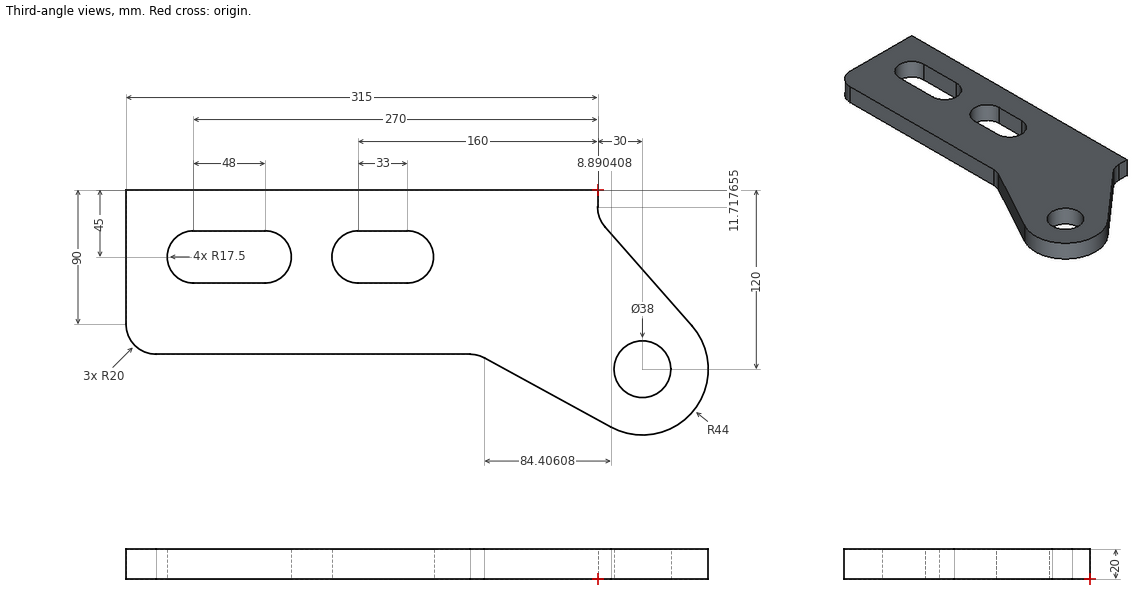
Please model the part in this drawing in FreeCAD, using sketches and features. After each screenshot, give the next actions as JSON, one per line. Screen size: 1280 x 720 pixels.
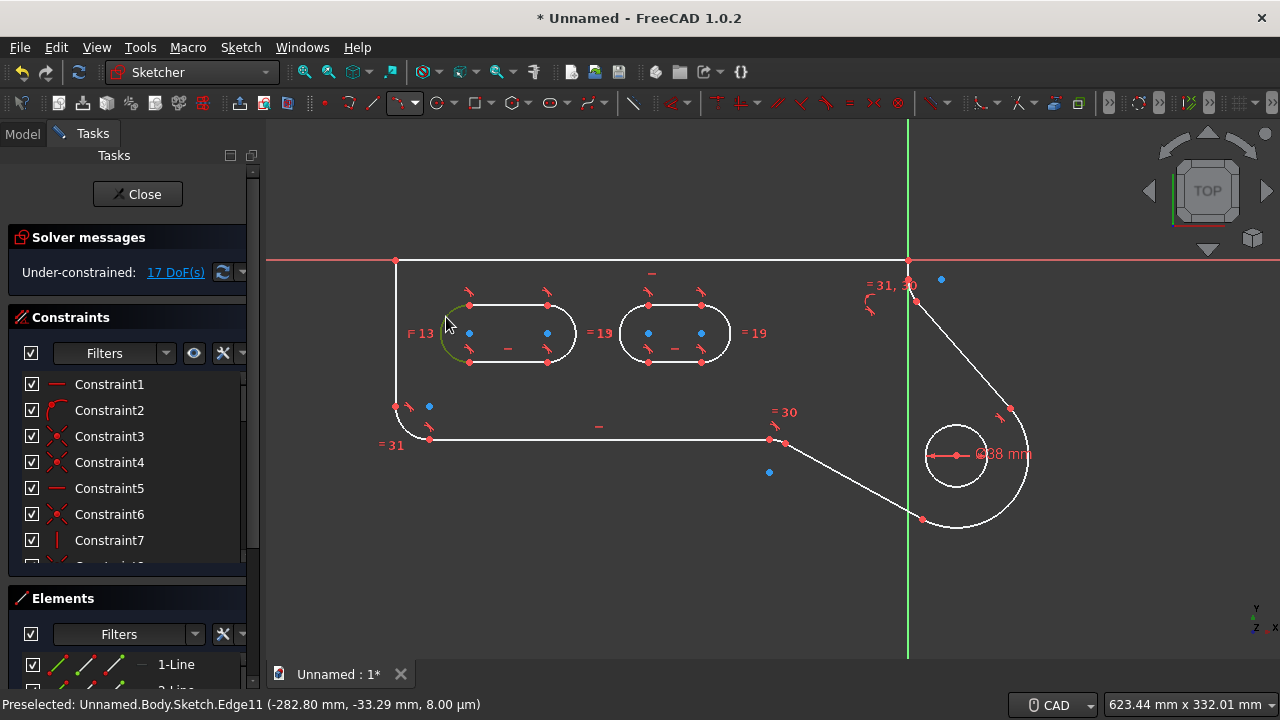
{"action": "left_click", "coordinate": [625, 317]}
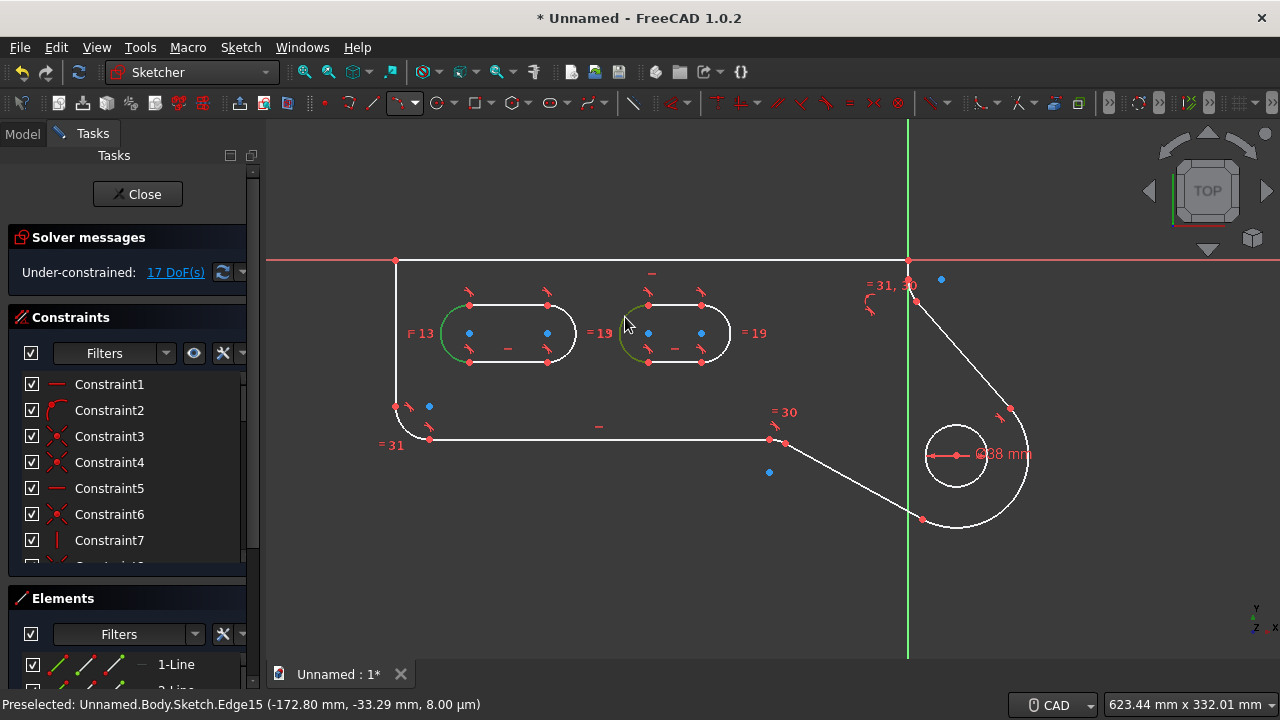
{"action": "left_click", "coordinate": [850, 104]}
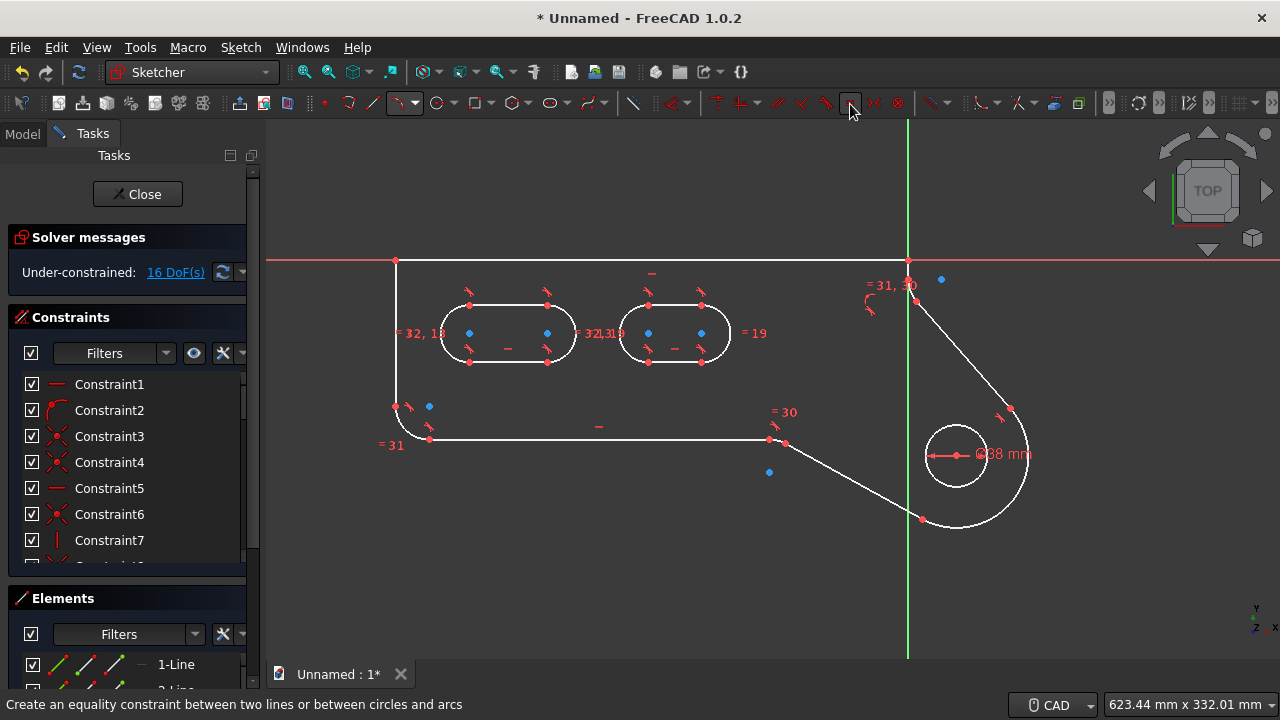
{"action": "scroll", "coordinate": [778, 441], "scroll_direction": "up", "scroll_amount": 3}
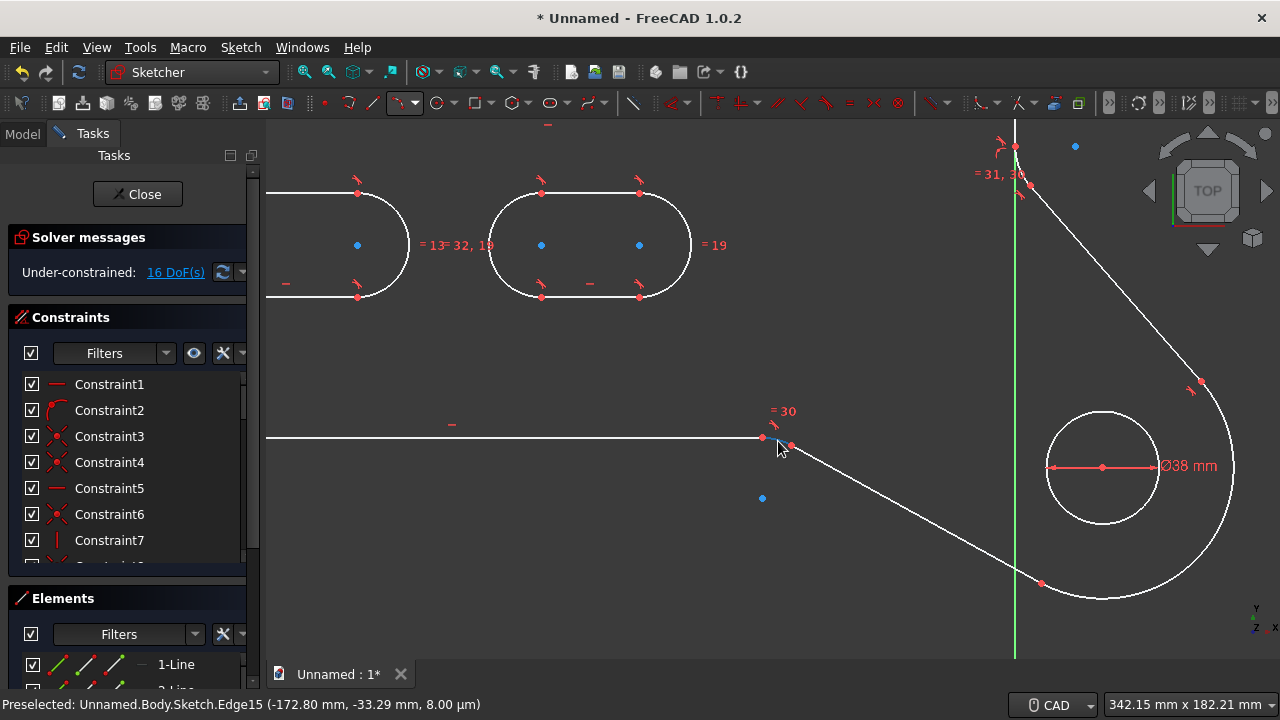
{"action": "left_click", "coordinate": [778, 440]}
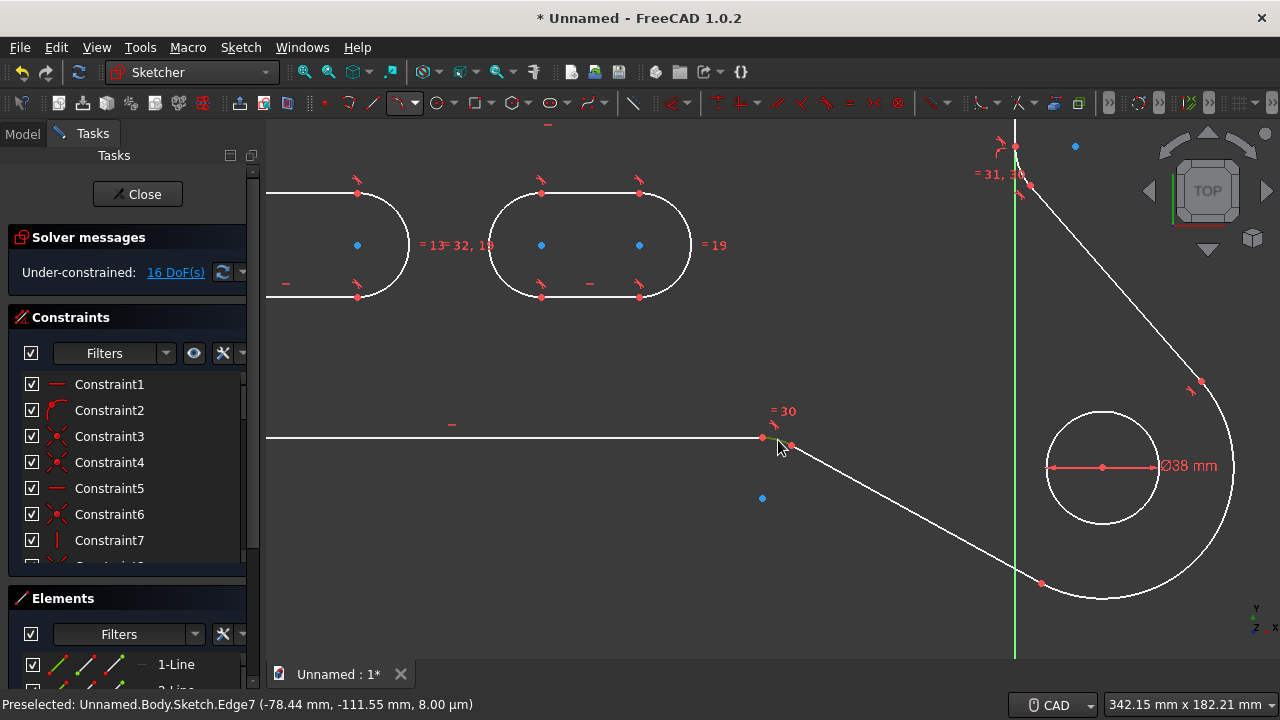
{"action": "key", "text": "k r"}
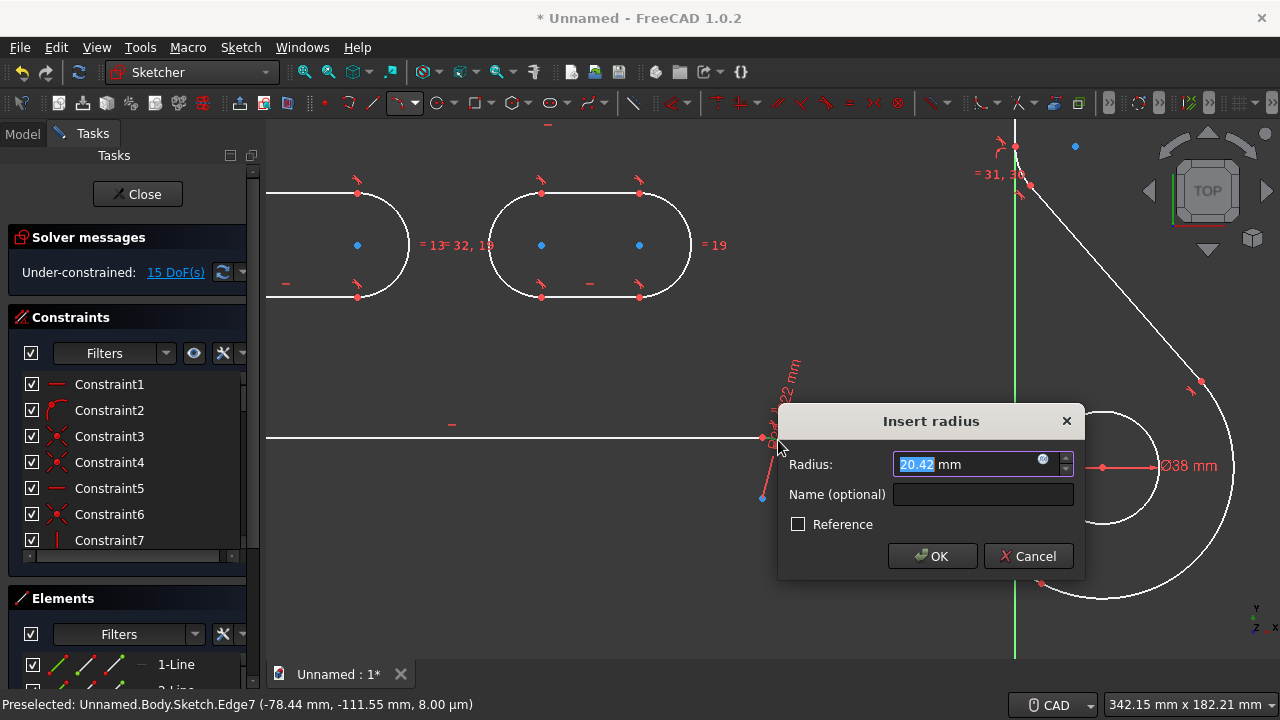
{"action": "type", "text": "20"}
{"action": "key", "text": "Return"}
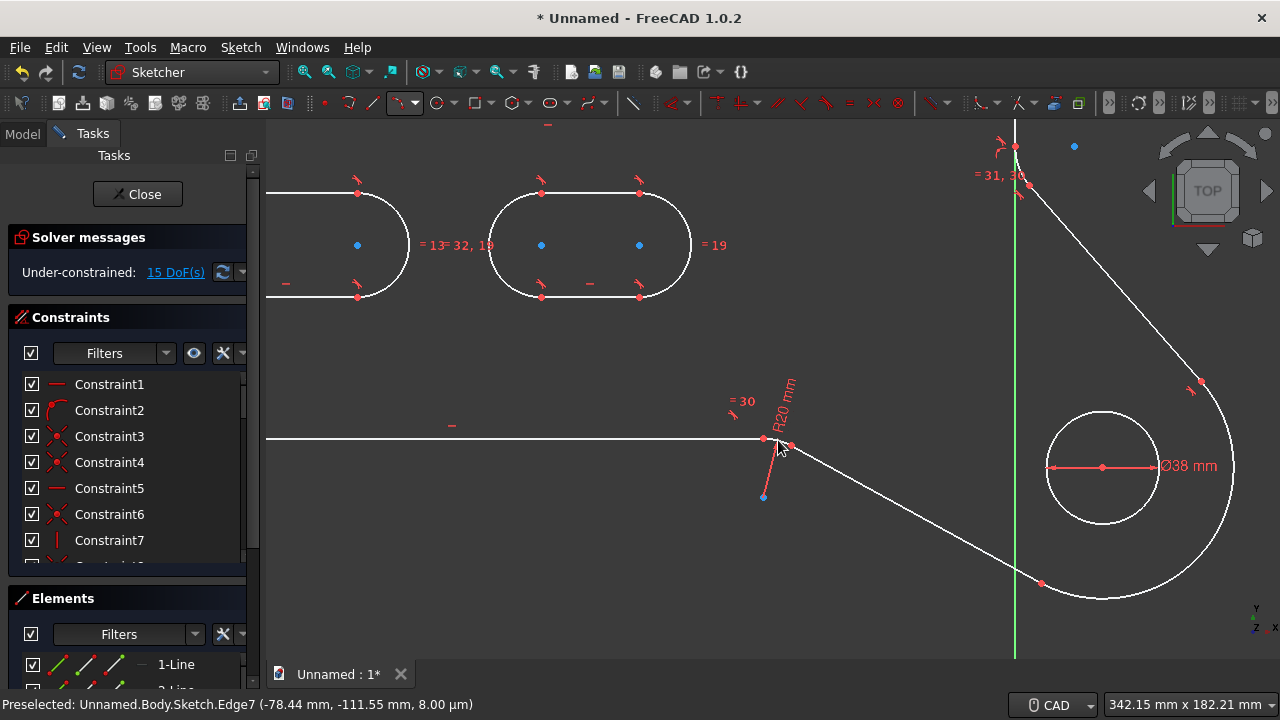
{"action": "left_click", "coordinate": [1111, 598]}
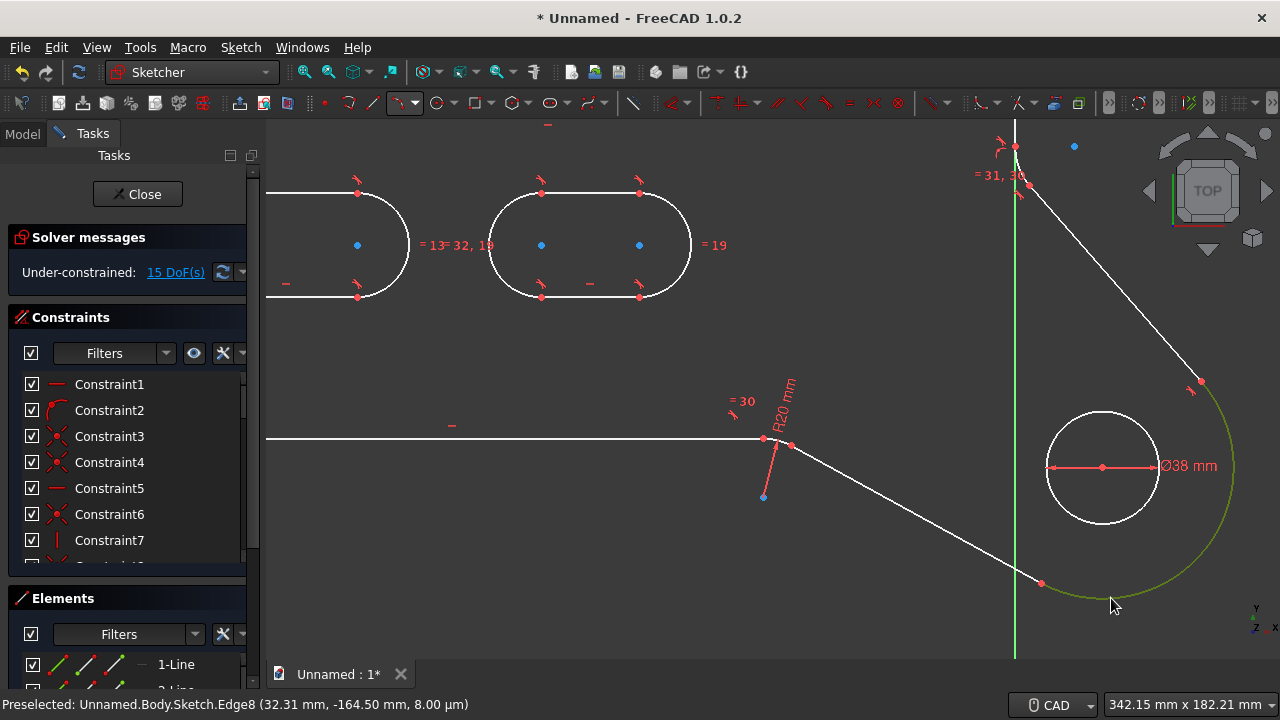
{"action": "left_click", "coordinate": [690, 104]}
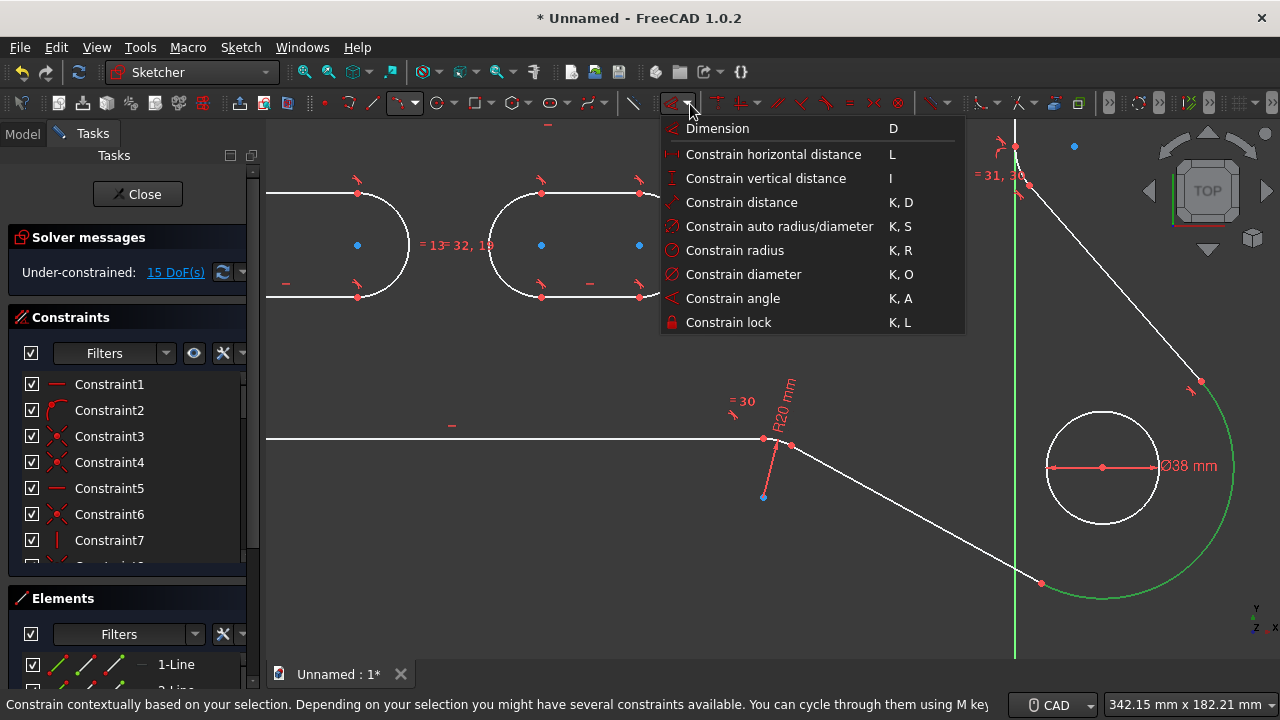
{"action": "left_click", "coordinate": [813, 250]}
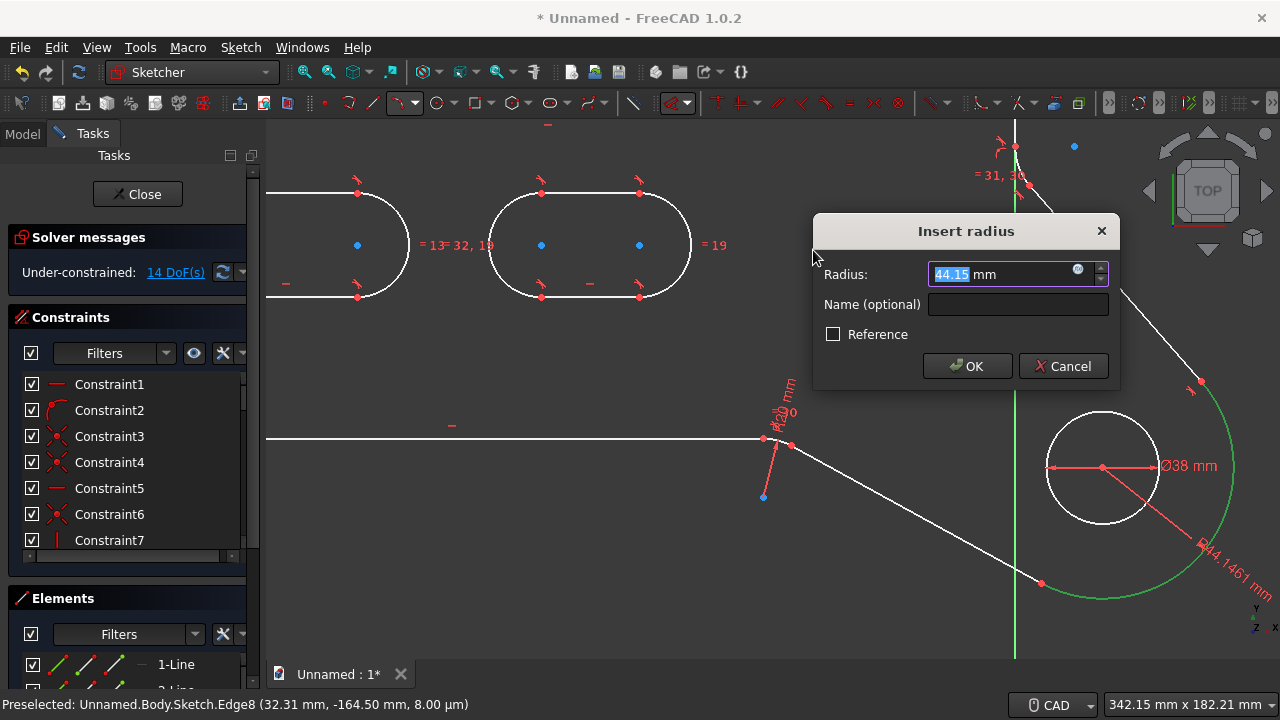
{"action": "type", "text": "44"}
{"action": "key", "text": "Return"}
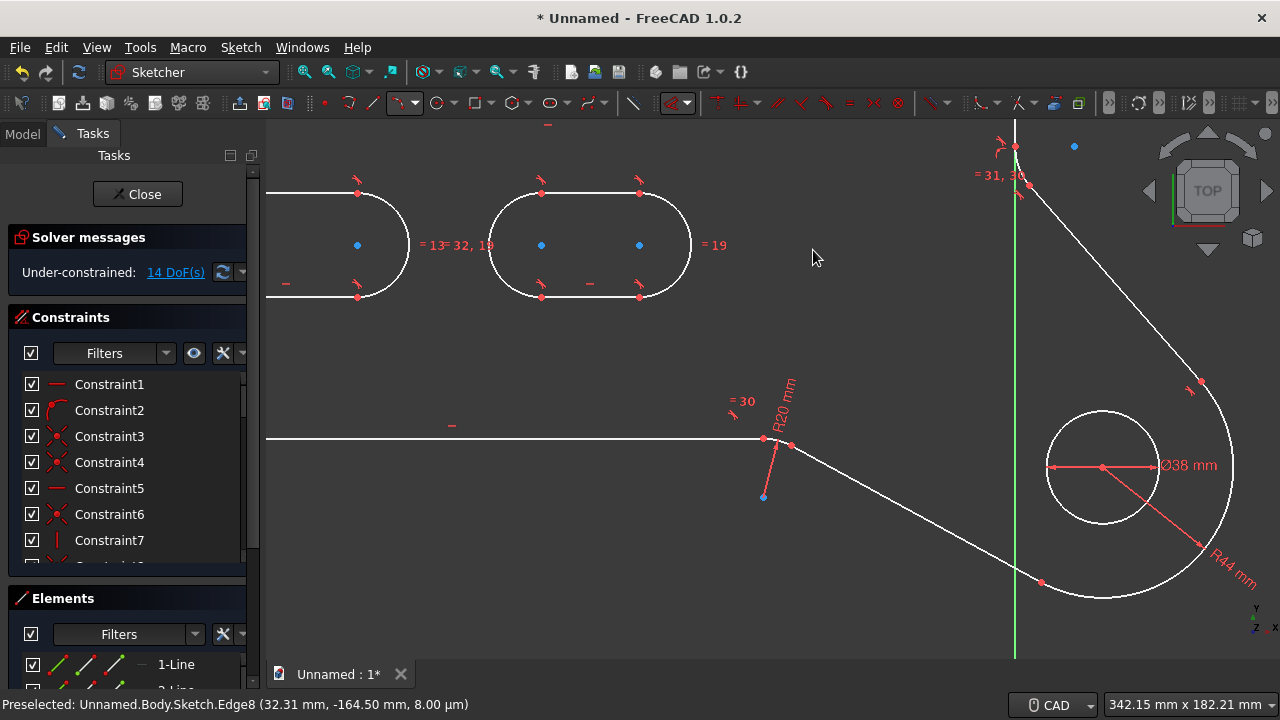
{"action": "scroll", "coordinate": [778, 441], "scroll_direction": "down", "scroll_amount": 3}